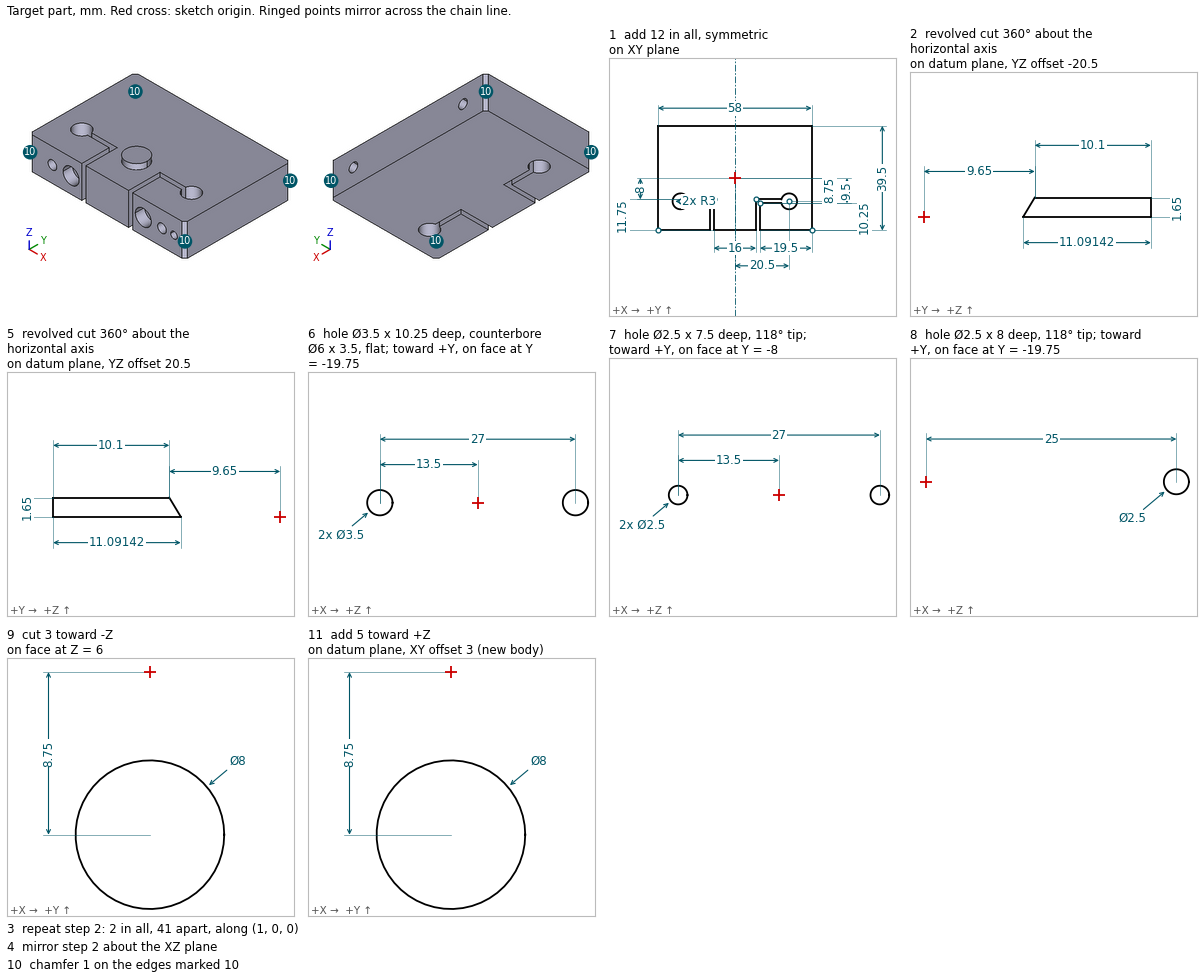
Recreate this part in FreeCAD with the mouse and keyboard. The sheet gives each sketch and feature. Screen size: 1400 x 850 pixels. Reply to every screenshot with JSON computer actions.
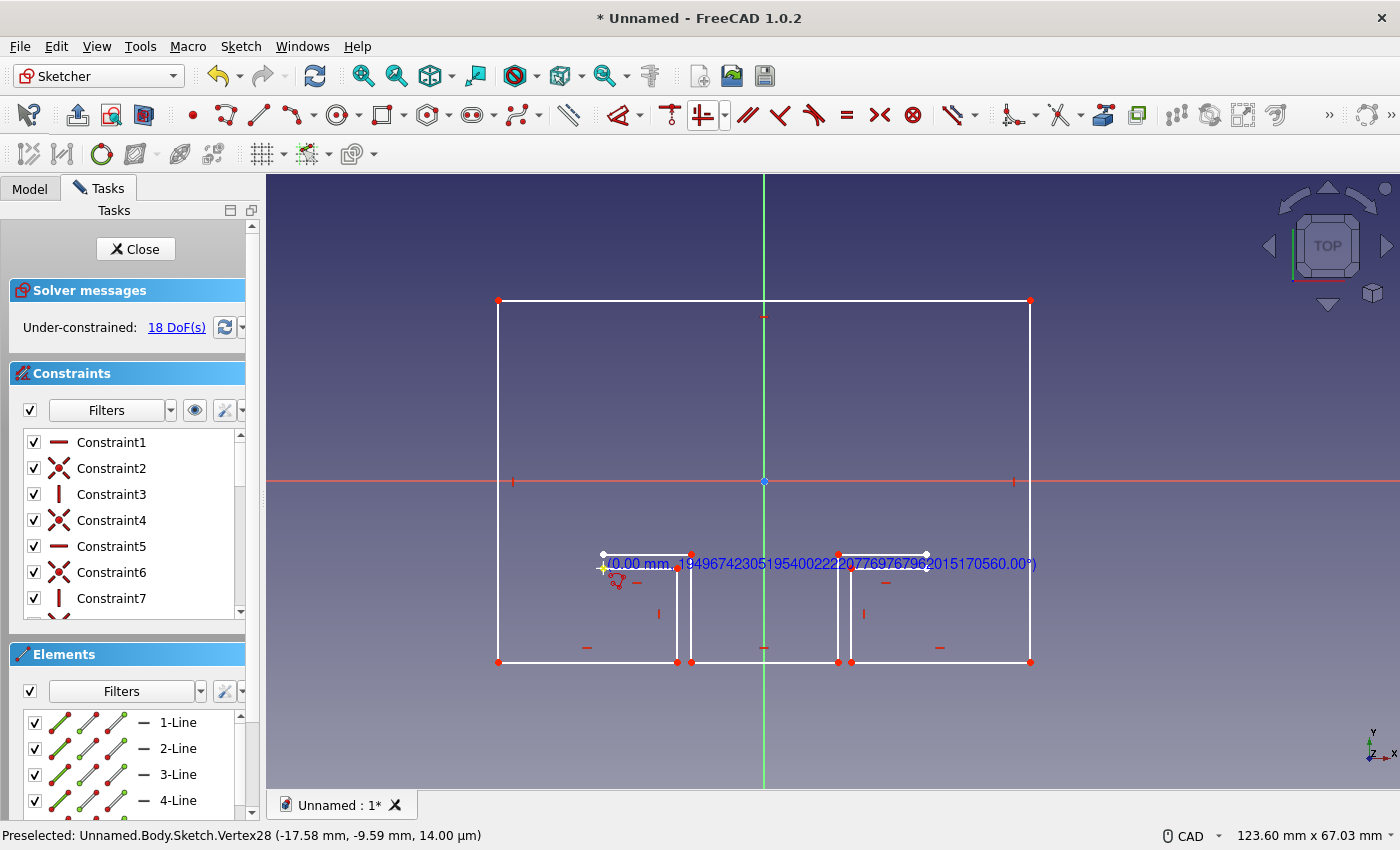
{"action": "left_click", "coordinate": [292, 116]}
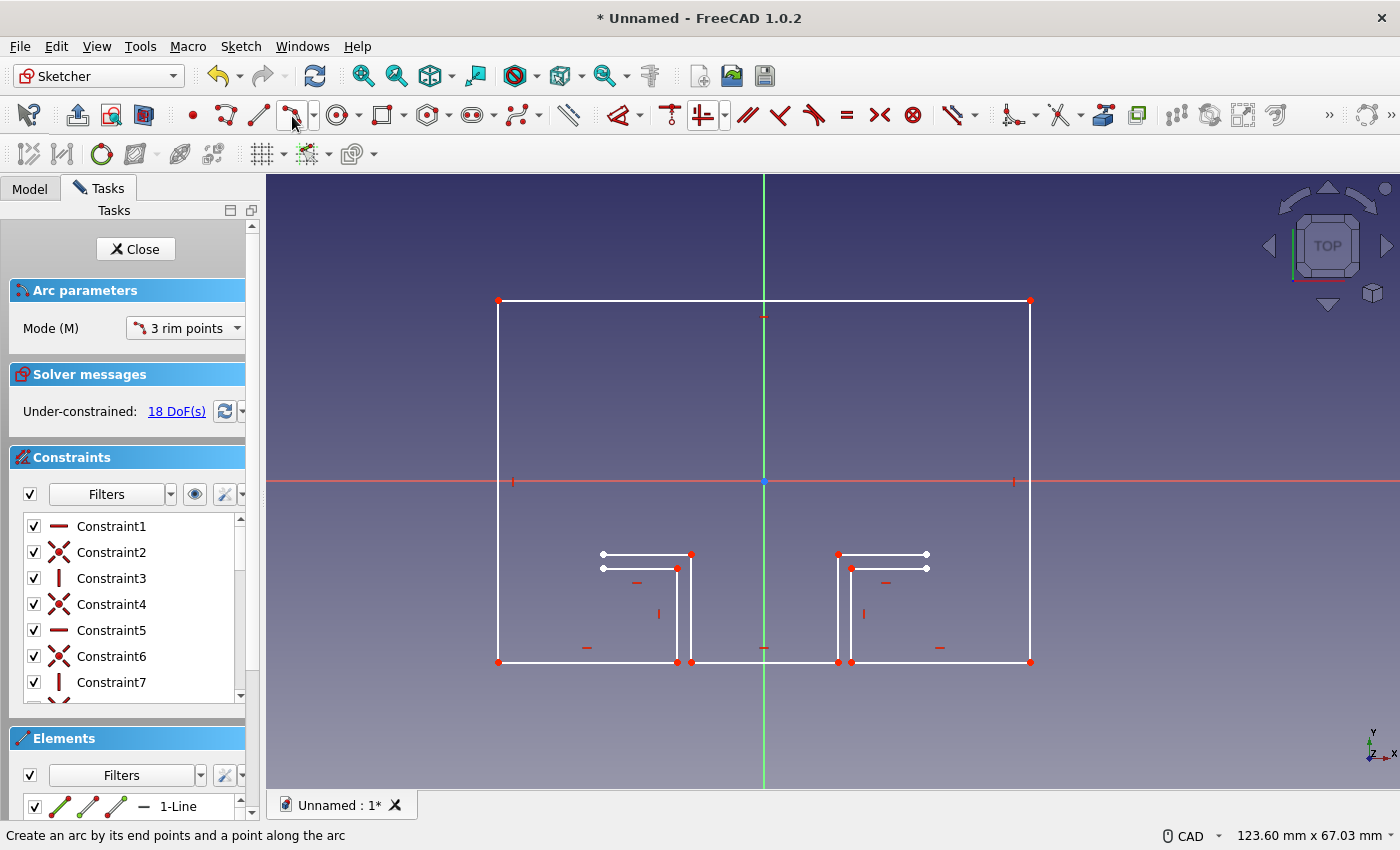
{"action": "left_click", "coordinate": [926, 555]}
{"action": "left_click", "coordinate": [926, 569]}
{"action": "left_click", "coordinate": [980, 561]}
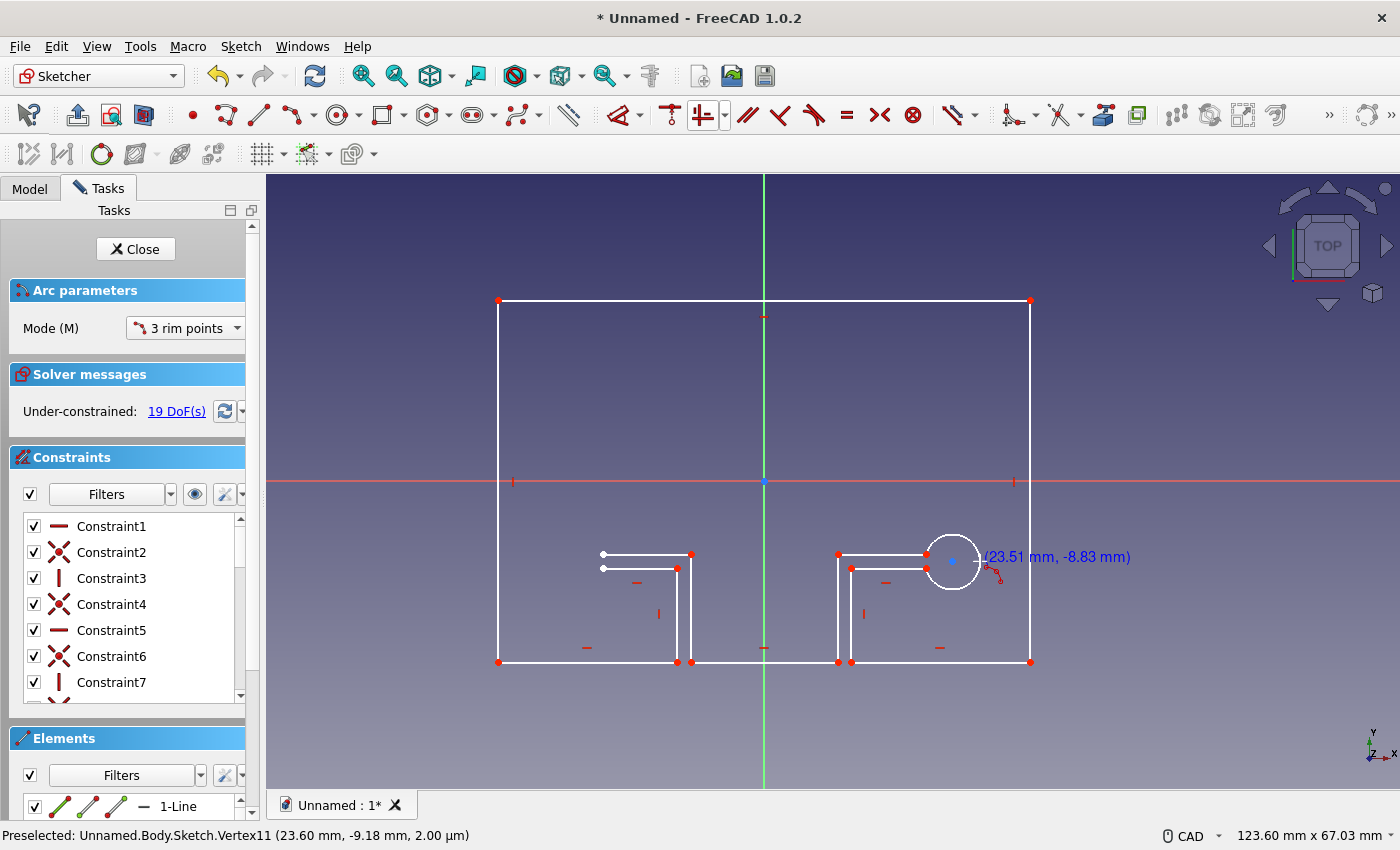
{"action": "left_click", "coordinate": [603, 569]}
{"action": "left_click", "coordinate": [603, 555]}
{"action": "left_click", "coordinate": [549, 561]}
{"action": "key", "text": "Escape"}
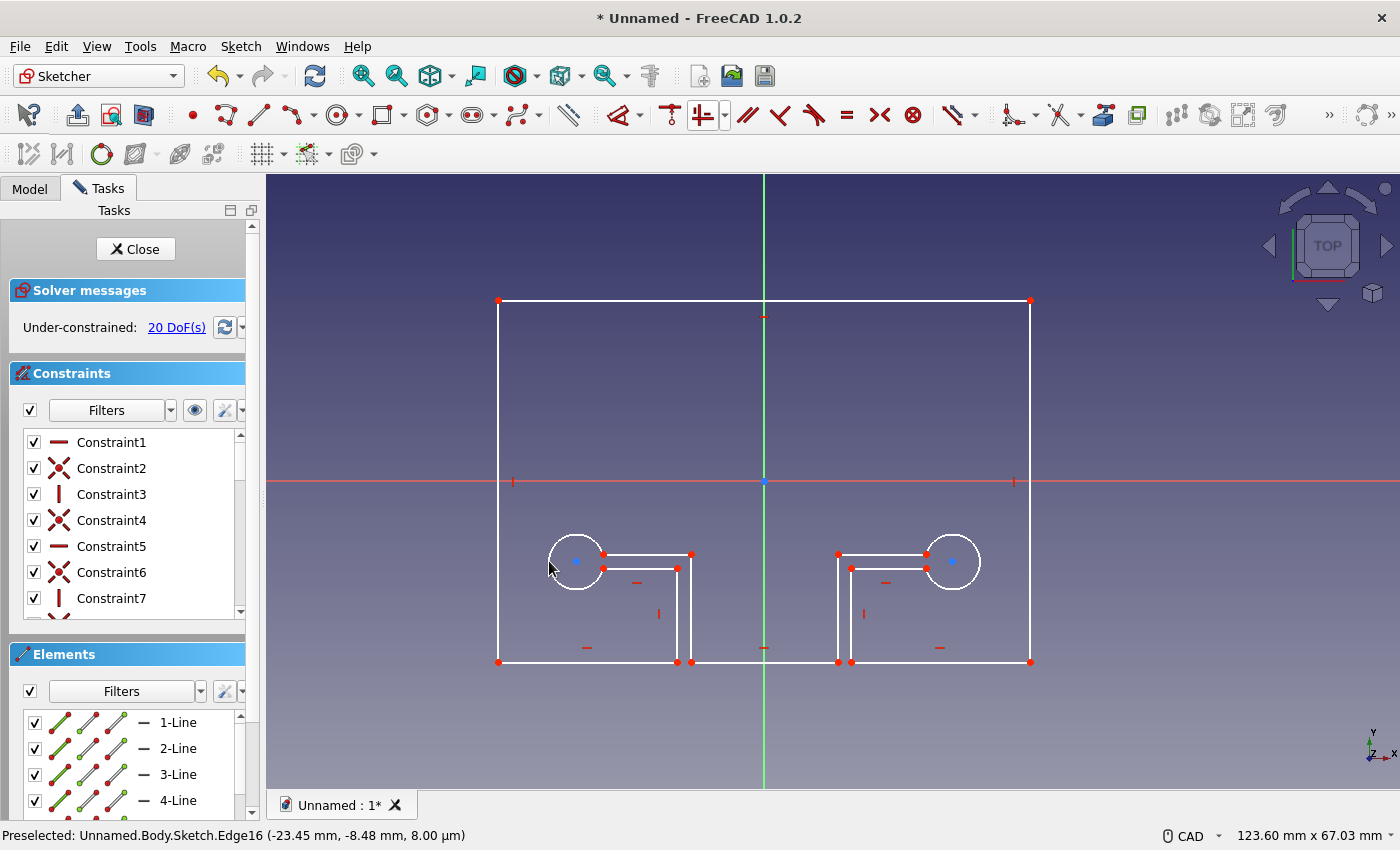
{"action": "left_click", "coordinate": [964, 587]}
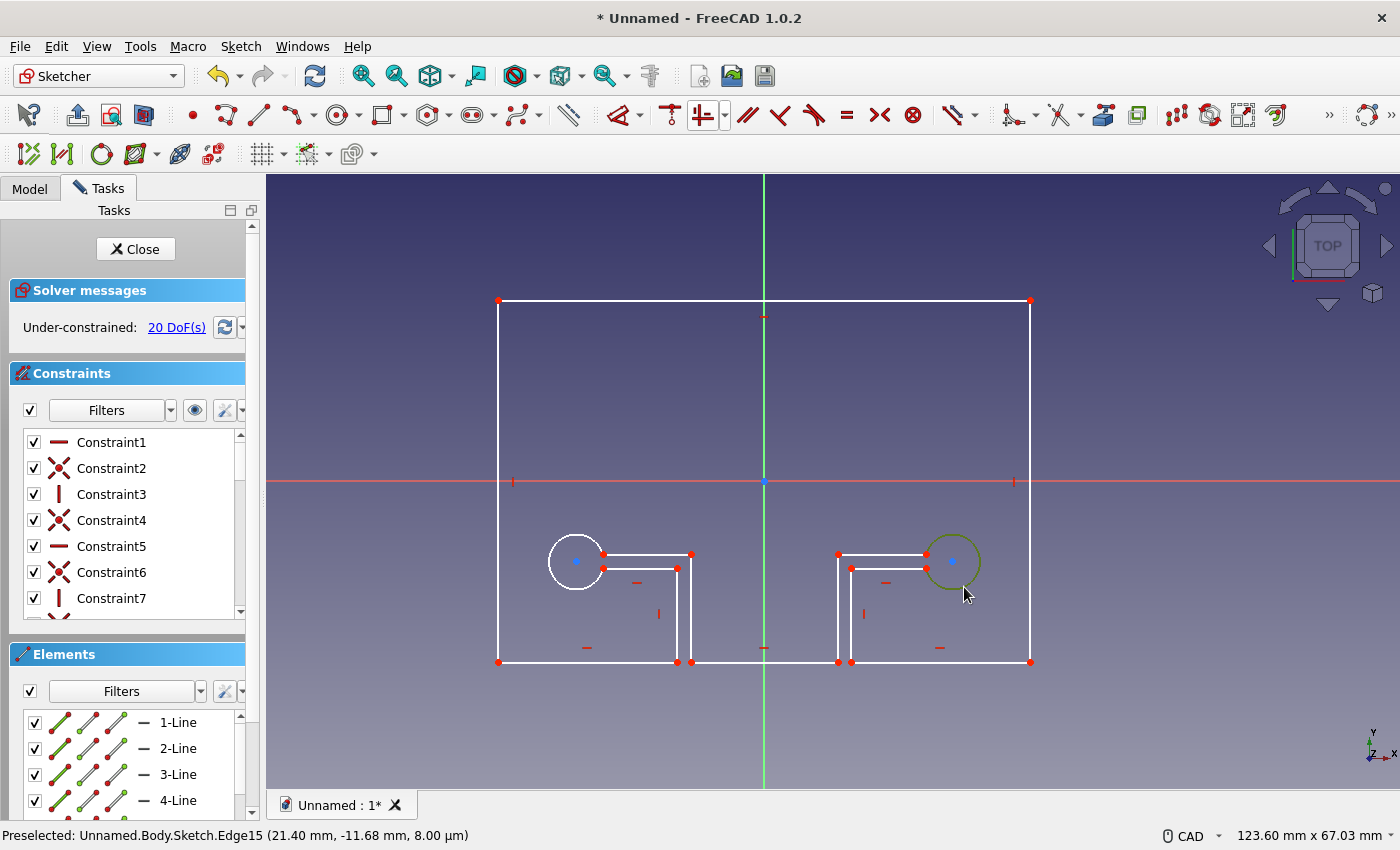
{"action": "left_click", "coordinate": [565, 537]}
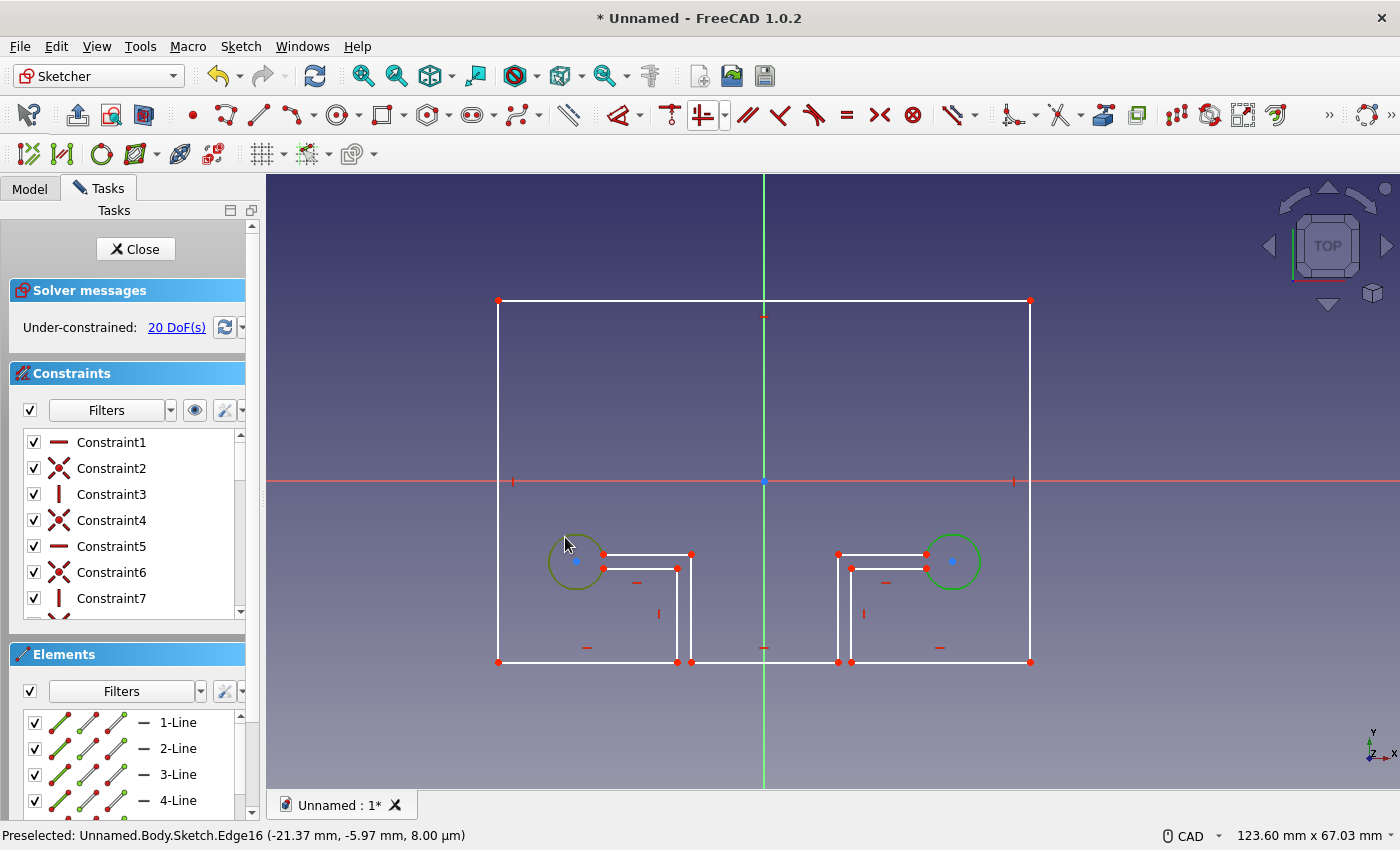
{"action": "left_click", "coordinate": [847, 116]}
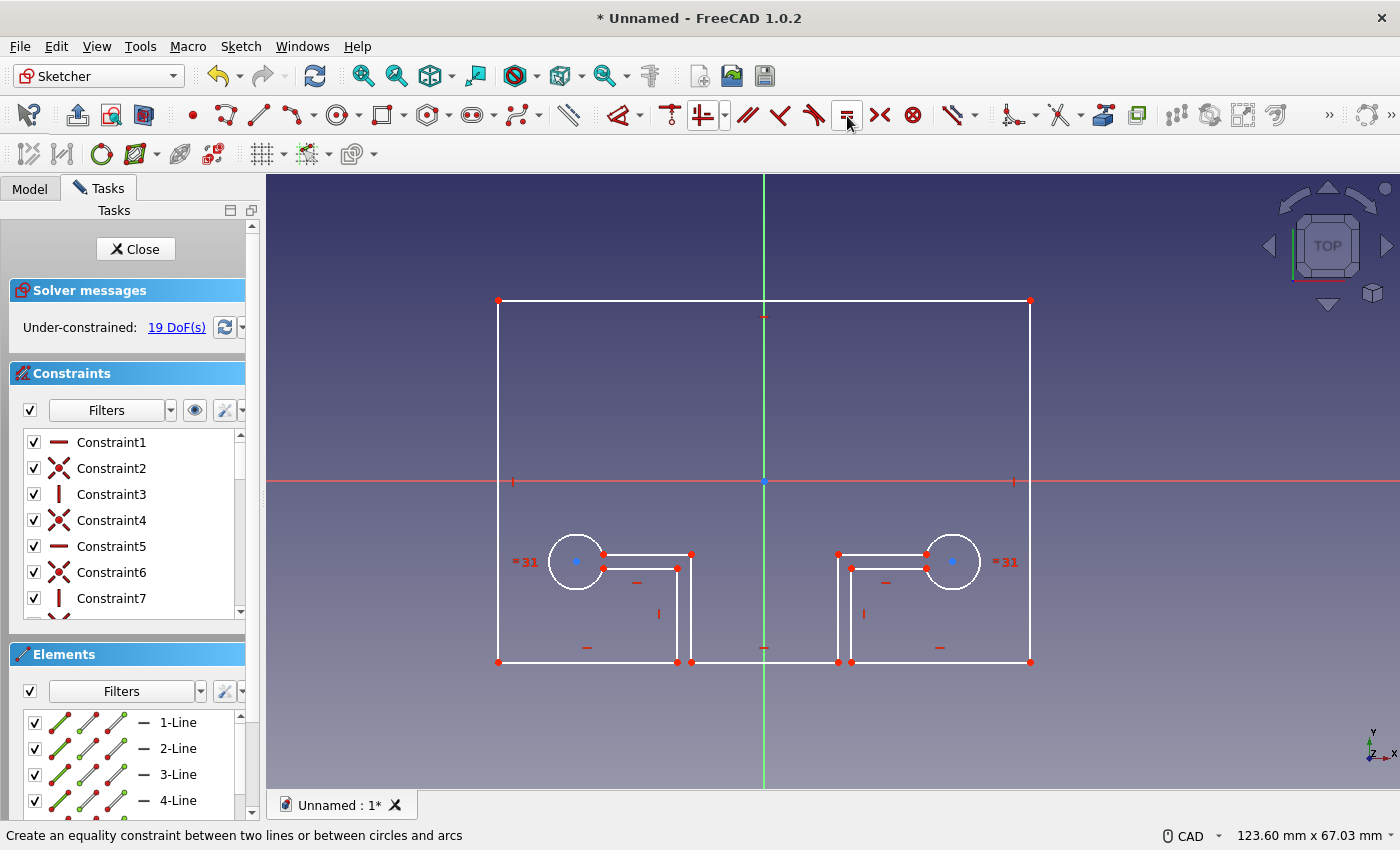
{"action": "left_click", "coordinate": [953, 562]}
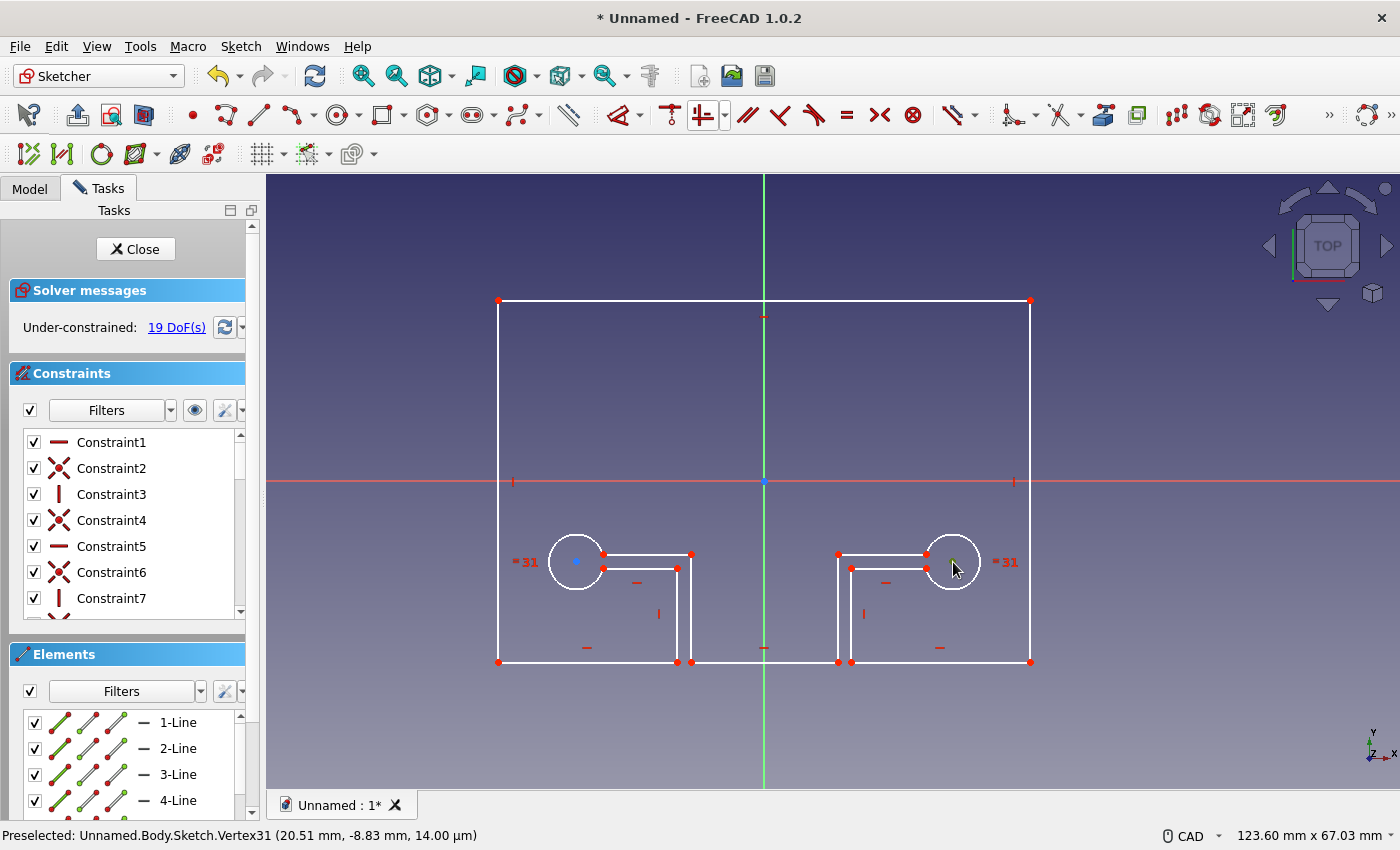
{"action": "left_click", "coordinate": [576, 562]}